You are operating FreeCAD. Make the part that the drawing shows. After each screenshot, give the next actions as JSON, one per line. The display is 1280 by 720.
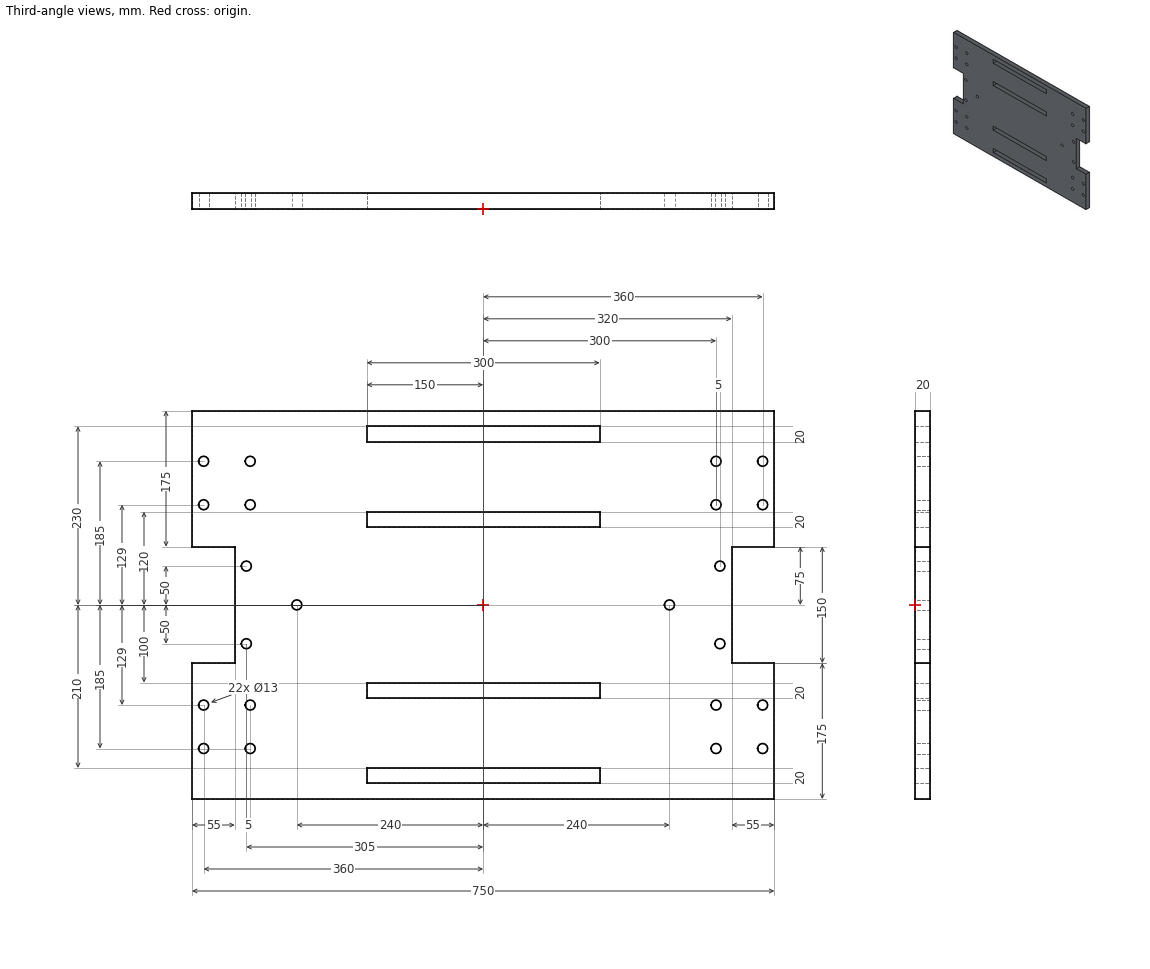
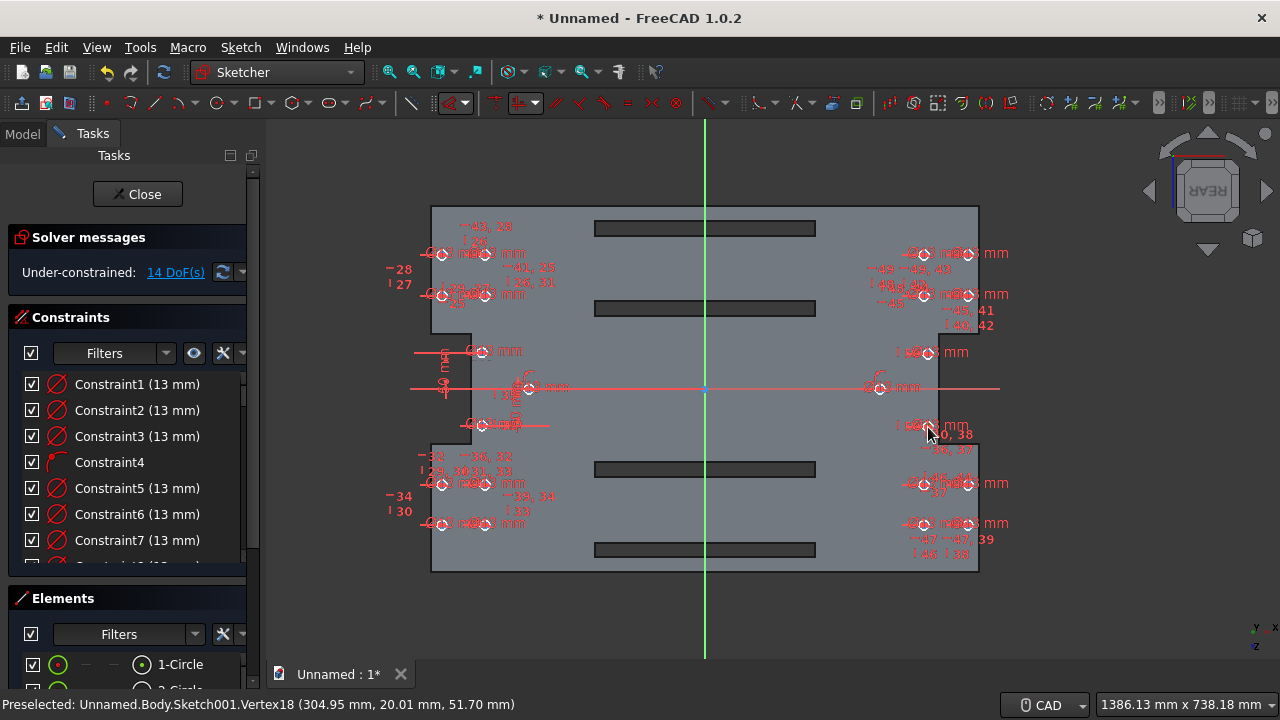
{"action": "key", "text": "i"}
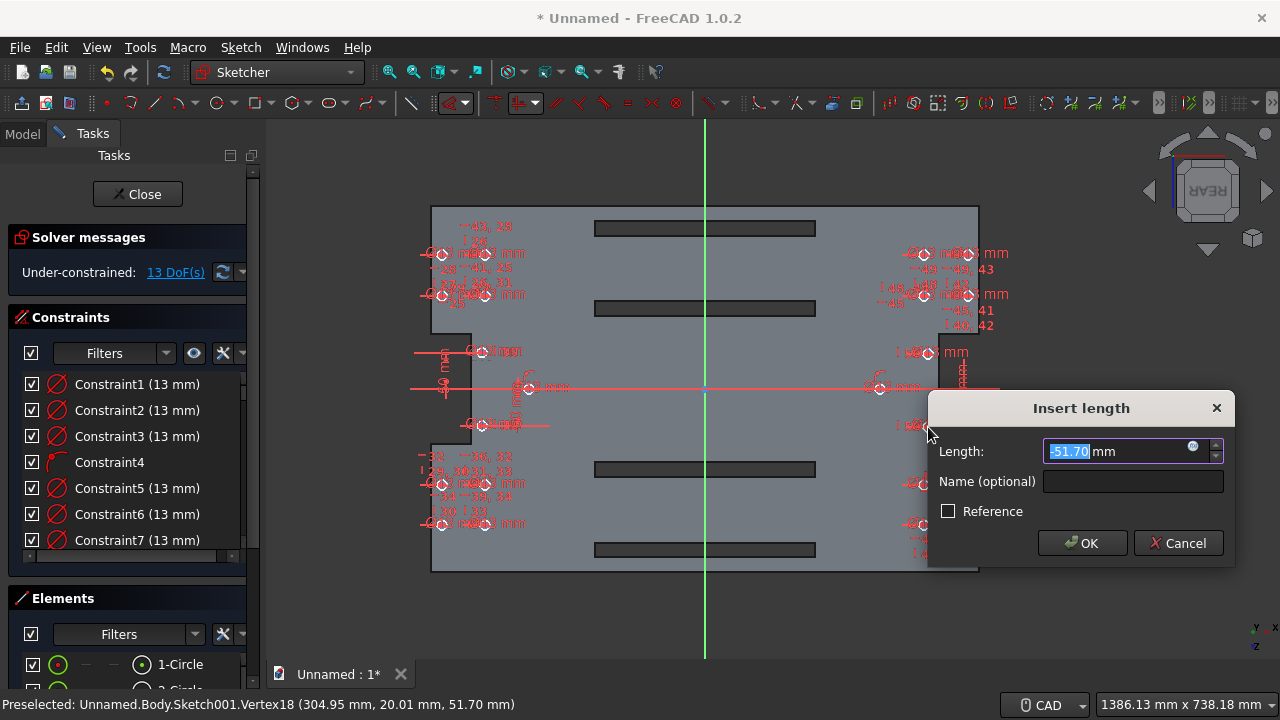
{"action": "type", "text": "-50"}
{"action": "key", "text": "Return"}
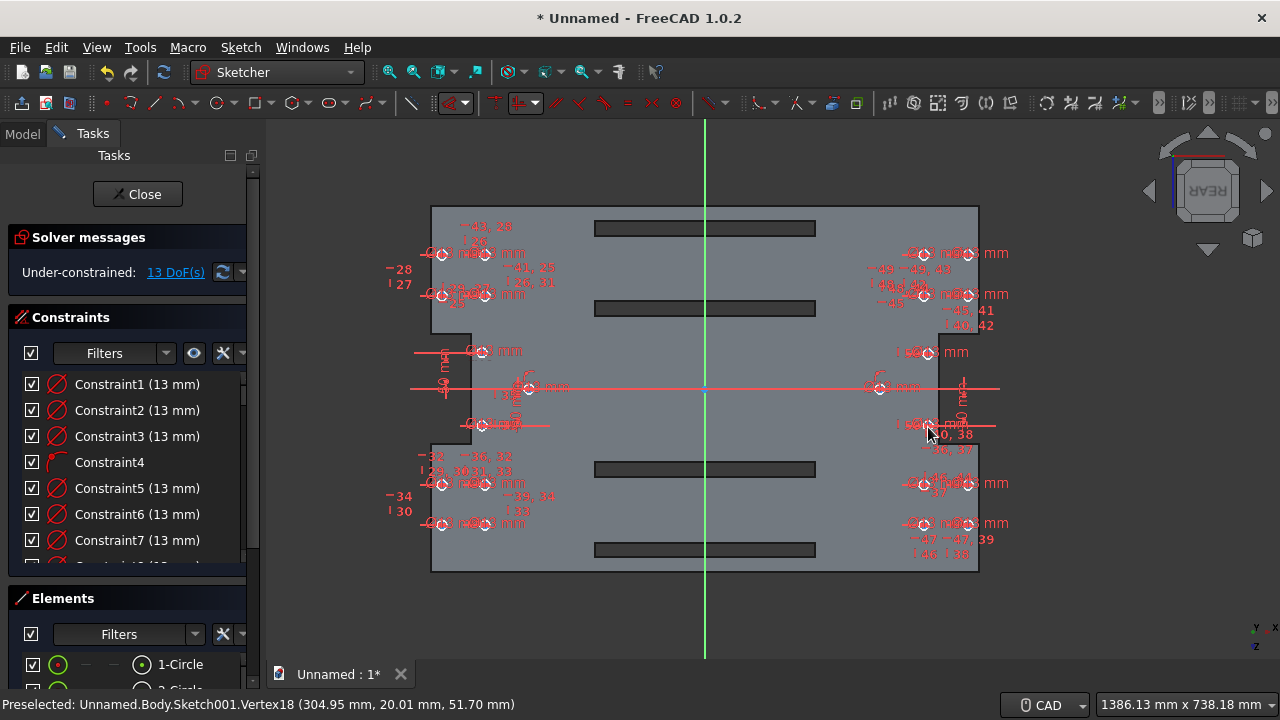
{"action": "left_click", "coordinate": [928, 354]}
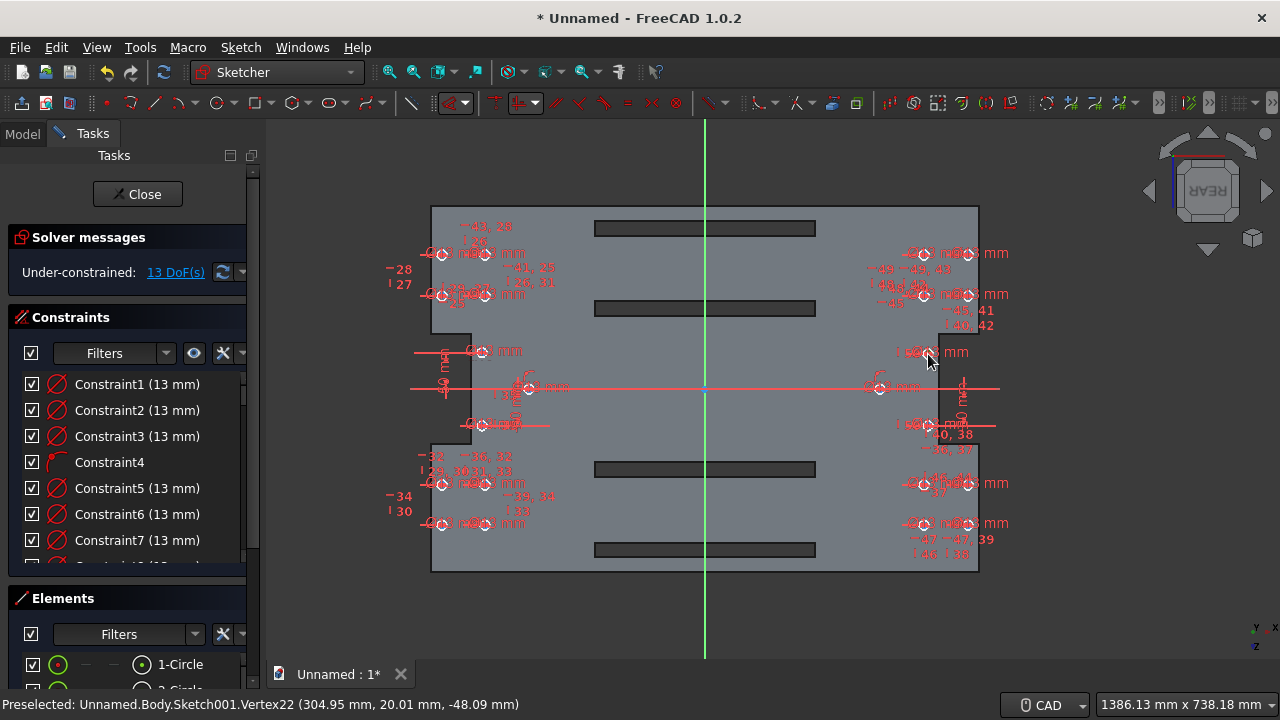
{"action": "key", "text": "i"}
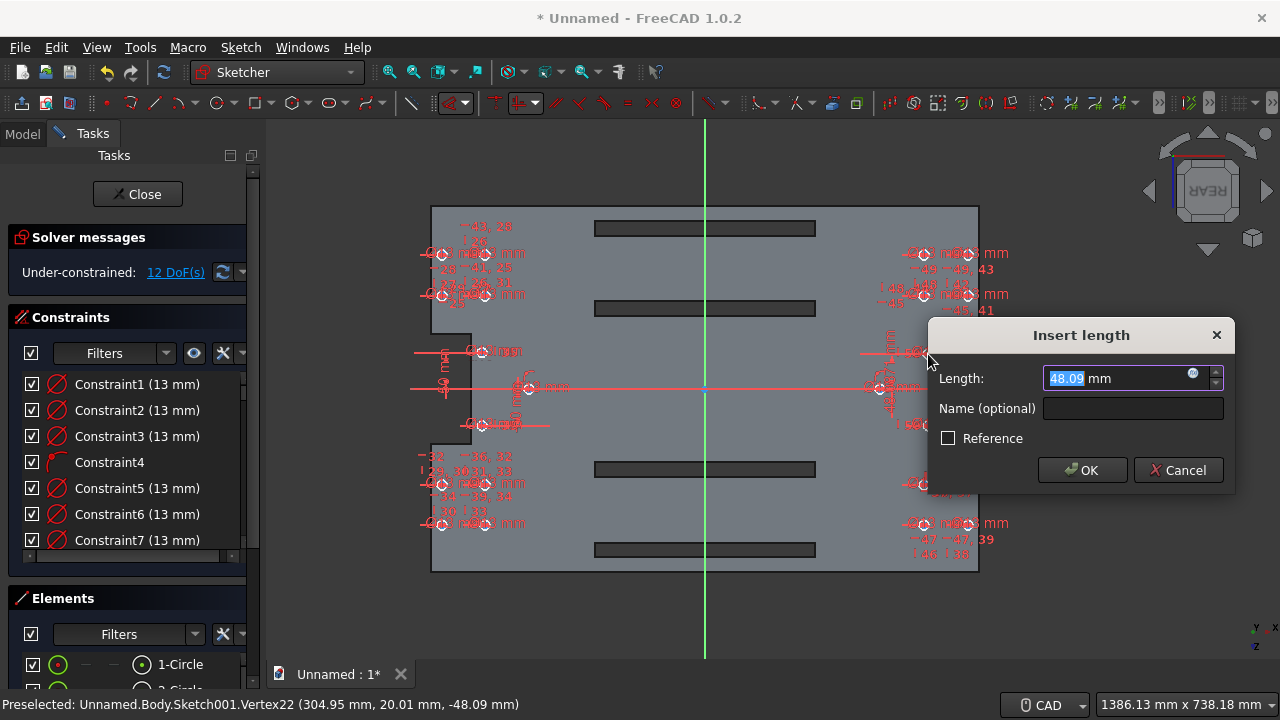
{"action": "type", "text": "50"}
{"action": "key", "text": "Return"}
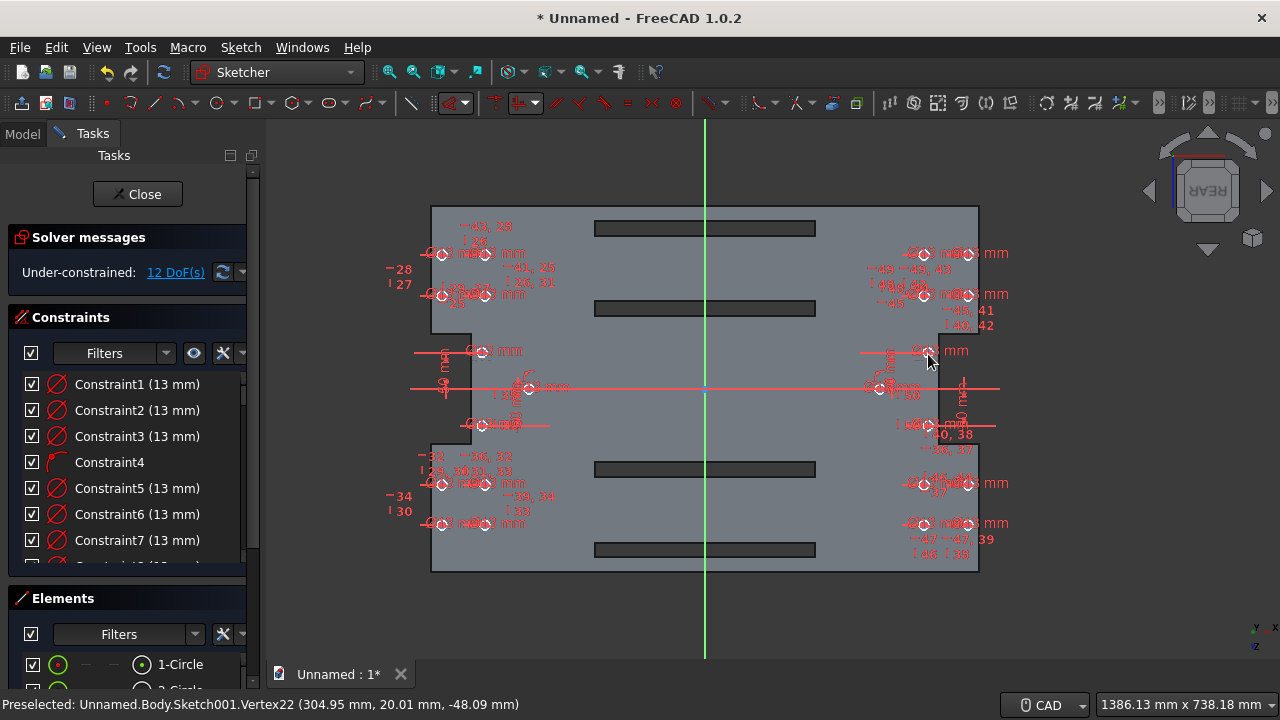
{"action": "scroll", "coordinate": [482, 353], "scroll_direction": "up", "scroll_amount": 12}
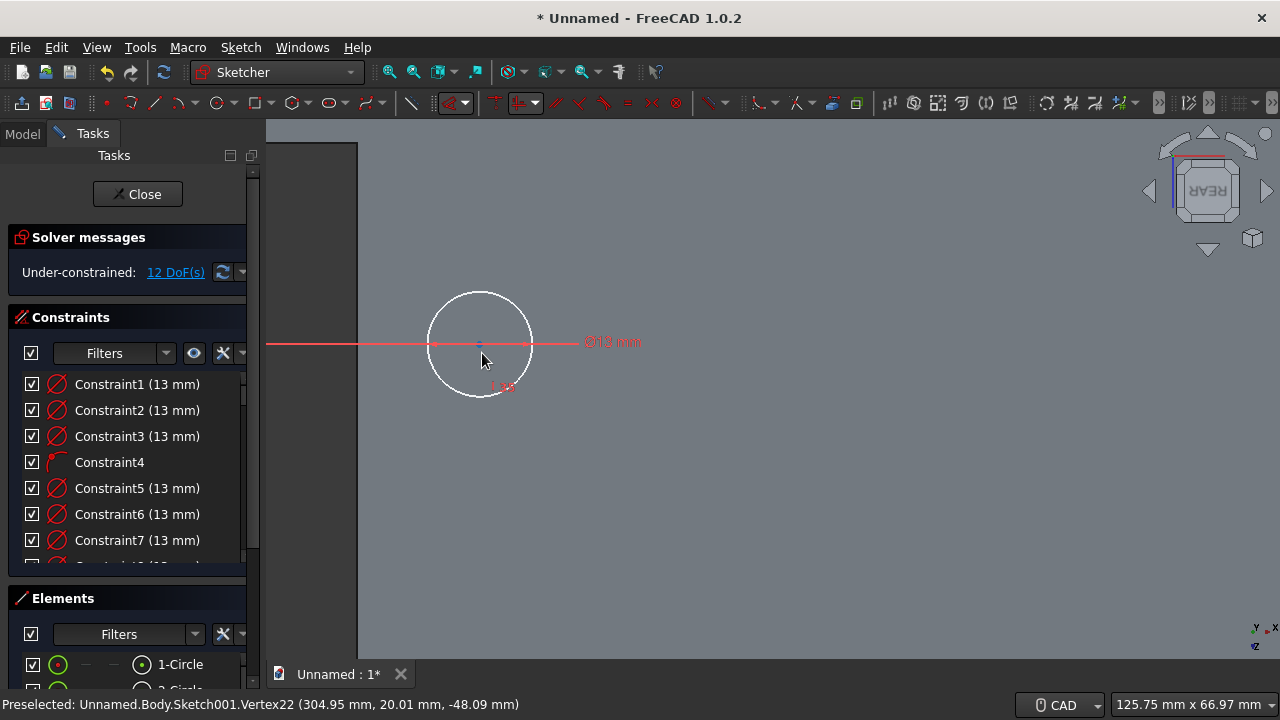
{"action": "left_click", "coordinate": [480, 344]}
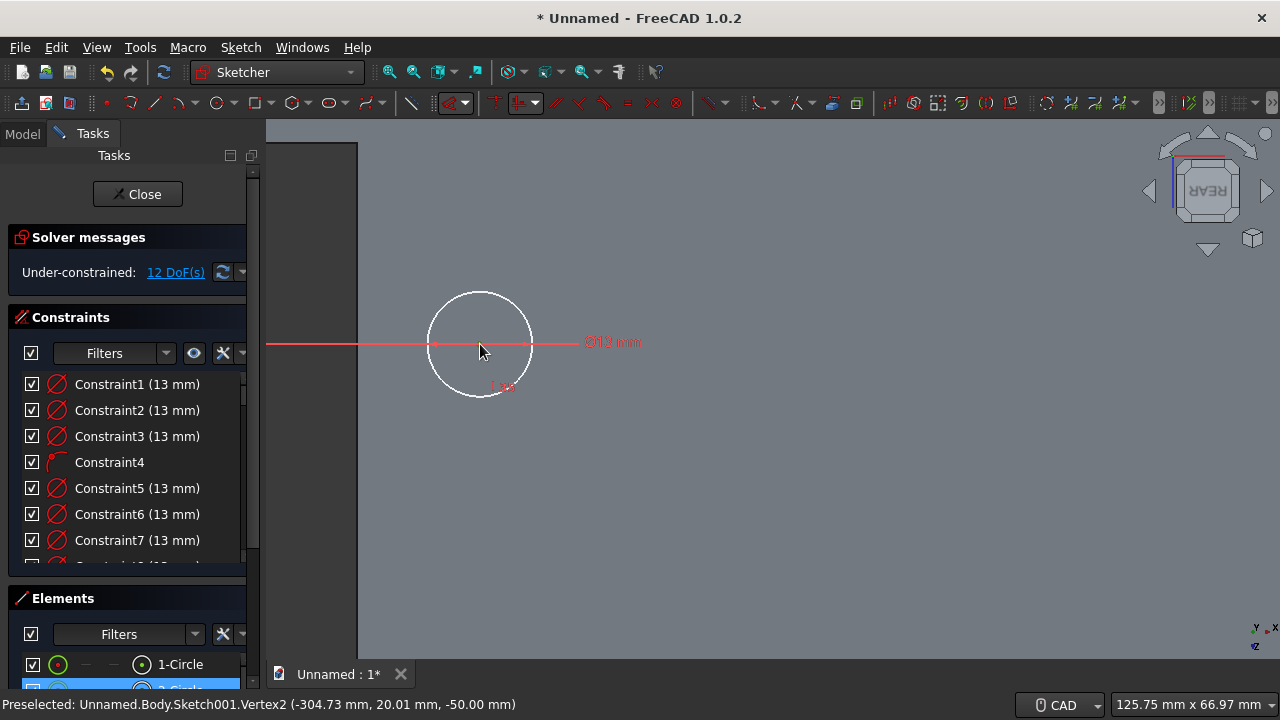
{"action": "scroll", "coordinate": [482, 353], "scroll_direction": "down", "scroll_amount": 12}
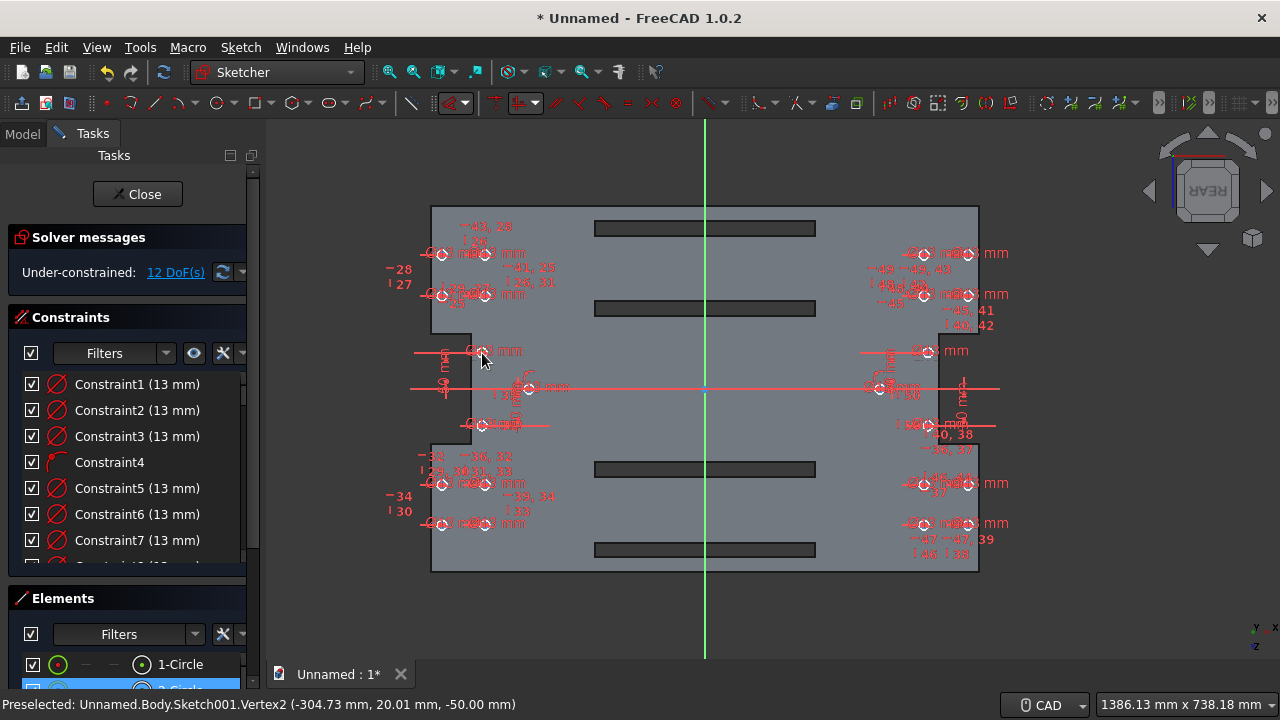
{"action": "scroll", "coordinate": [485, 296], "scroll_direction": "up", "scroll_amount": 12}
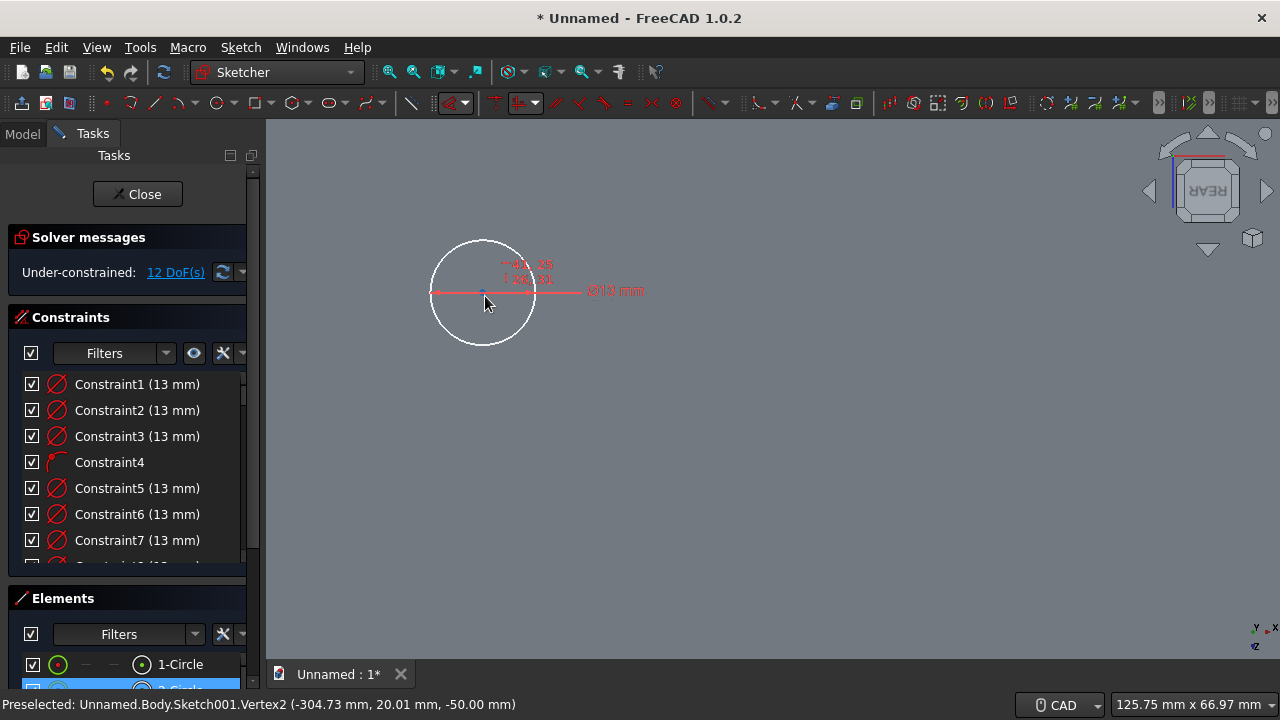
{"action": "left_click", "coordinate": [483, 293]}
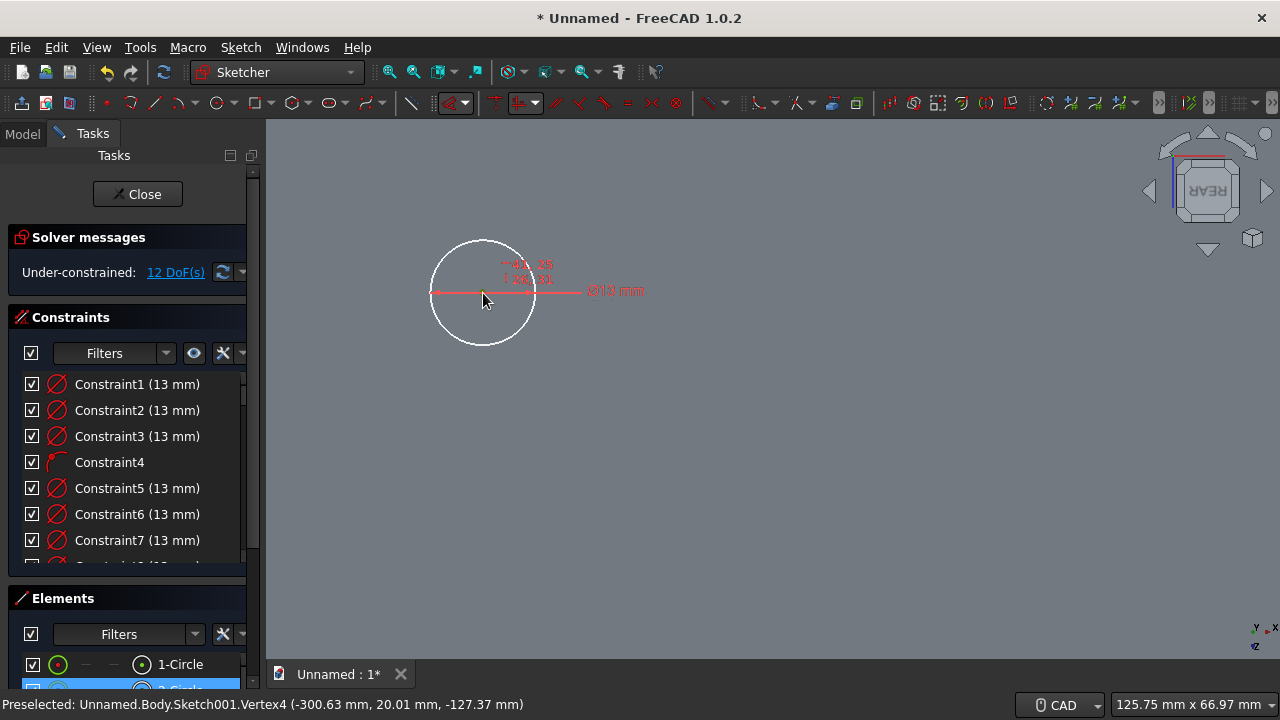
{"action": "key", "text": "l"}